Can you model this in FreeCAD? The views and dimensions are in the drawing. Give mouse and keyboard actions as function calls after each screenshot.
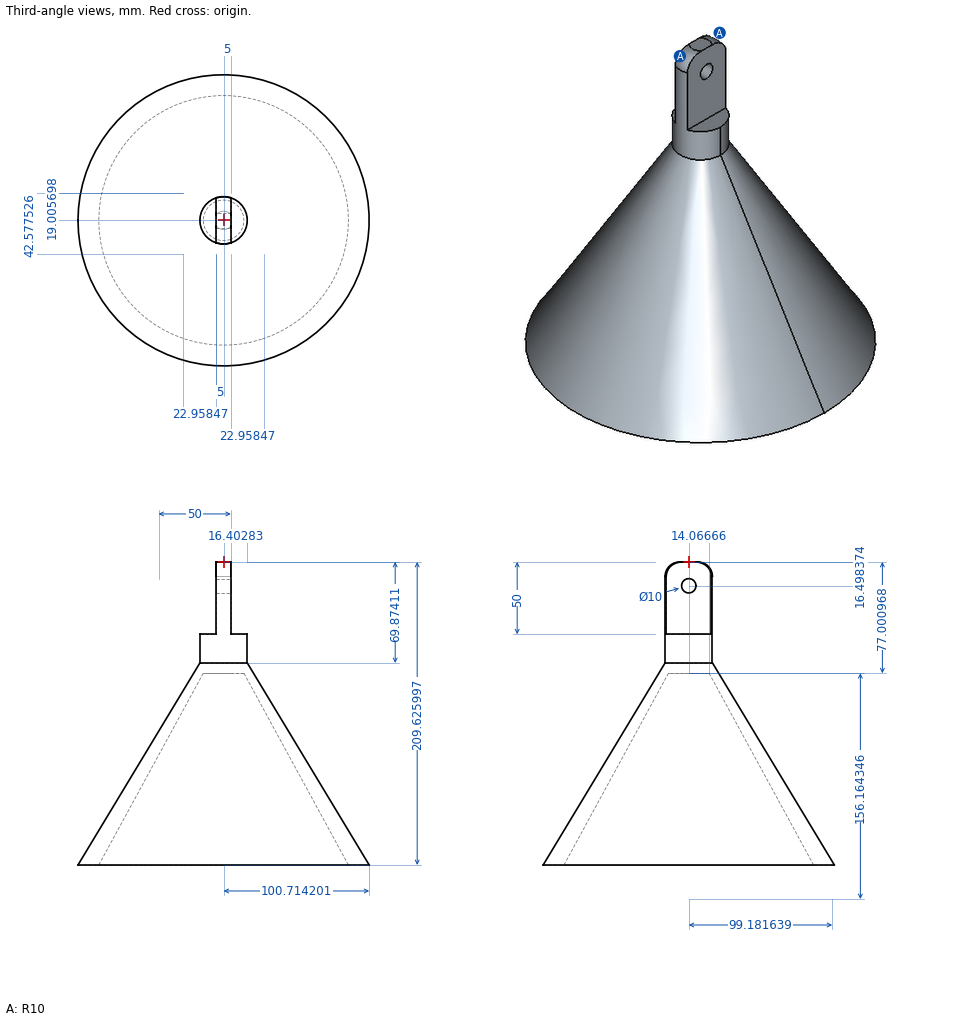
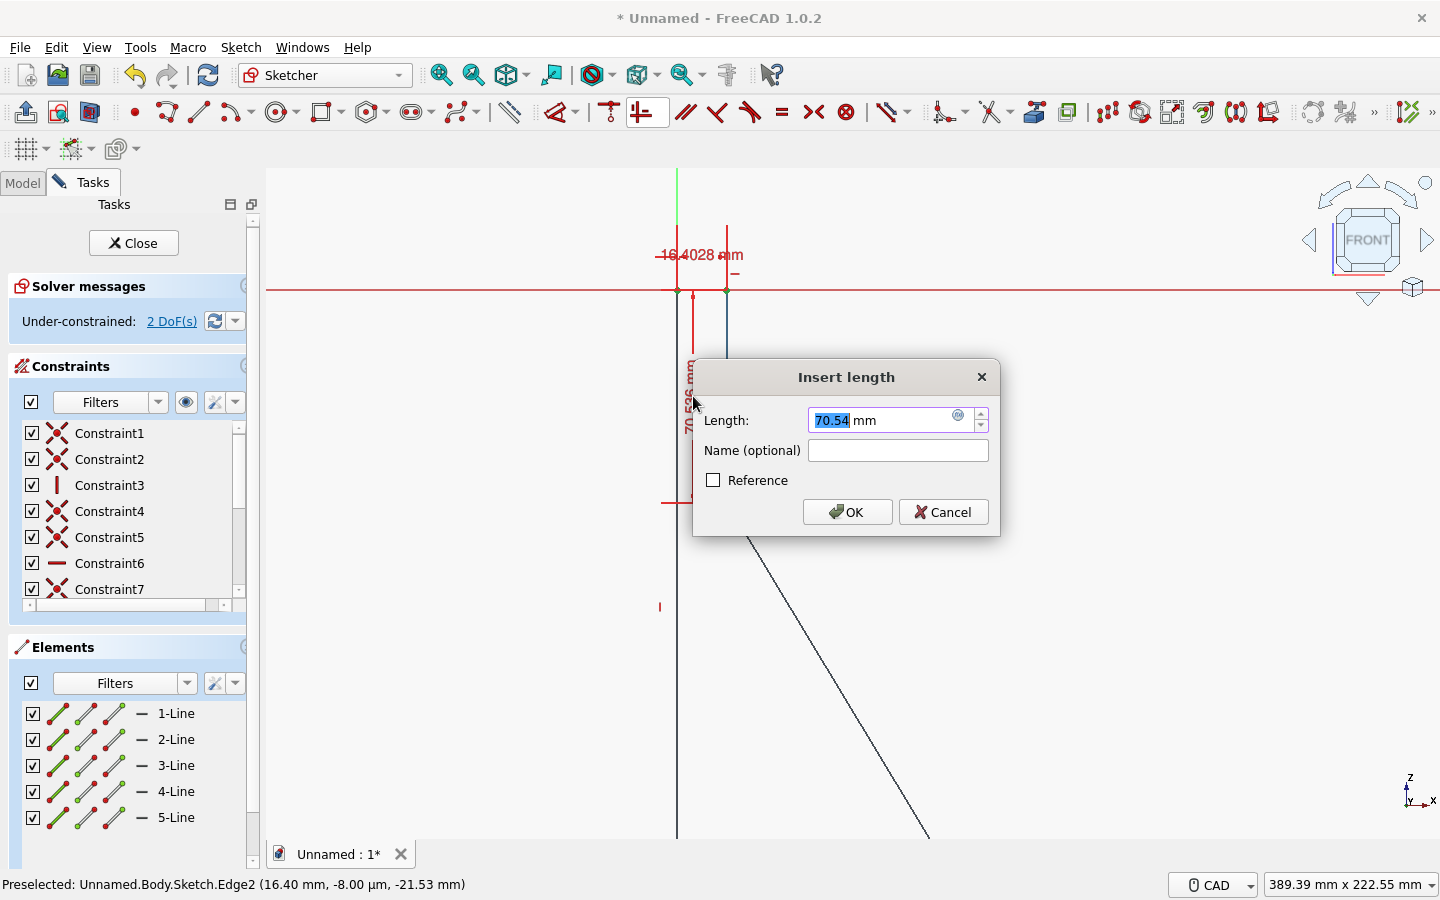
text(69.87411)
key(Return)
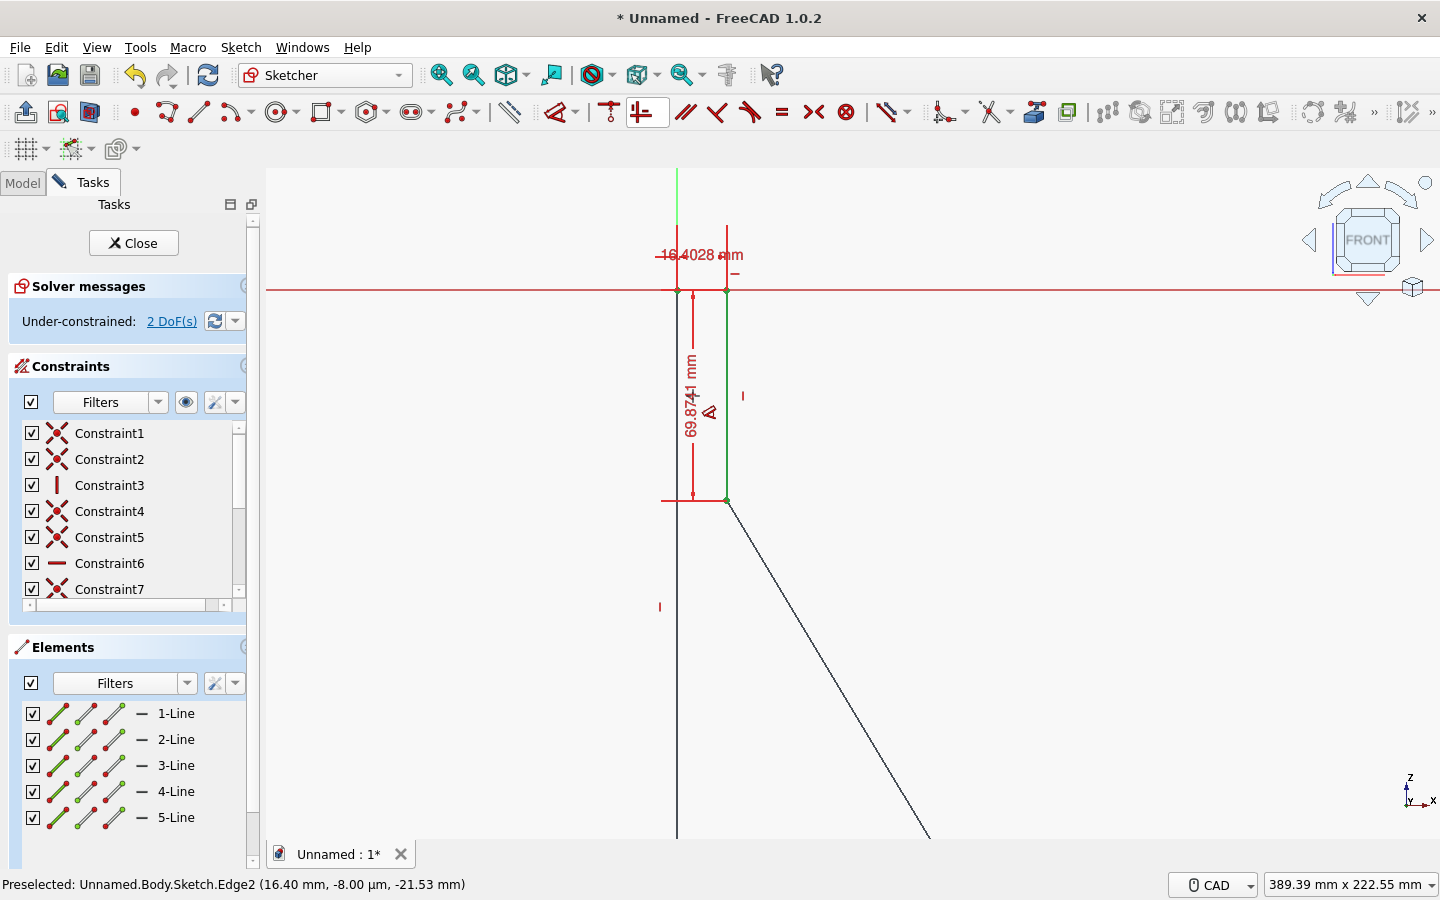
scroll(693, 295, down, 2)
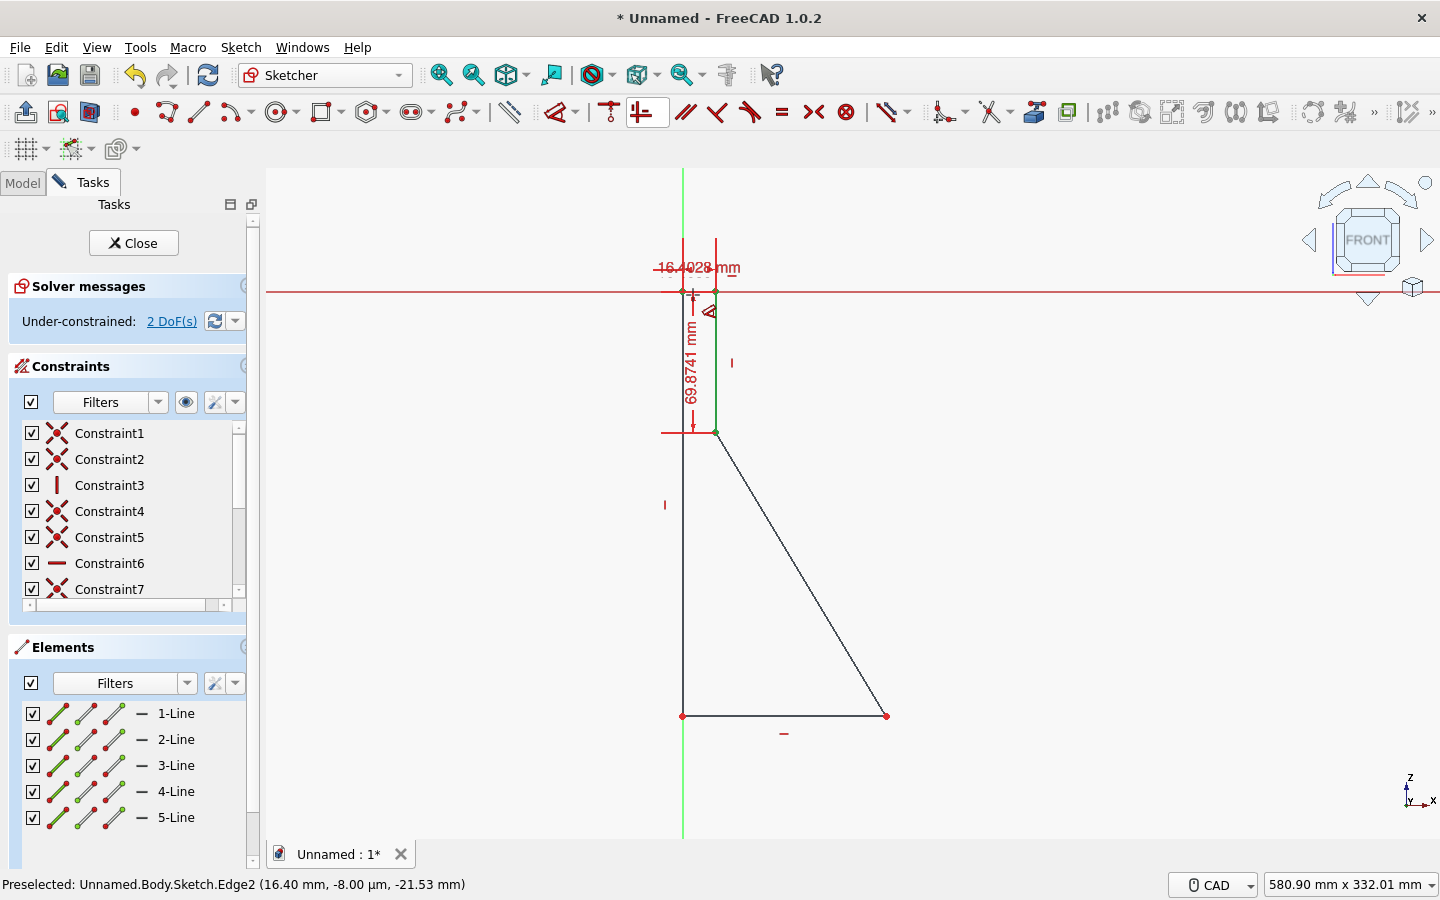
click(825, 716)
click(784, 750)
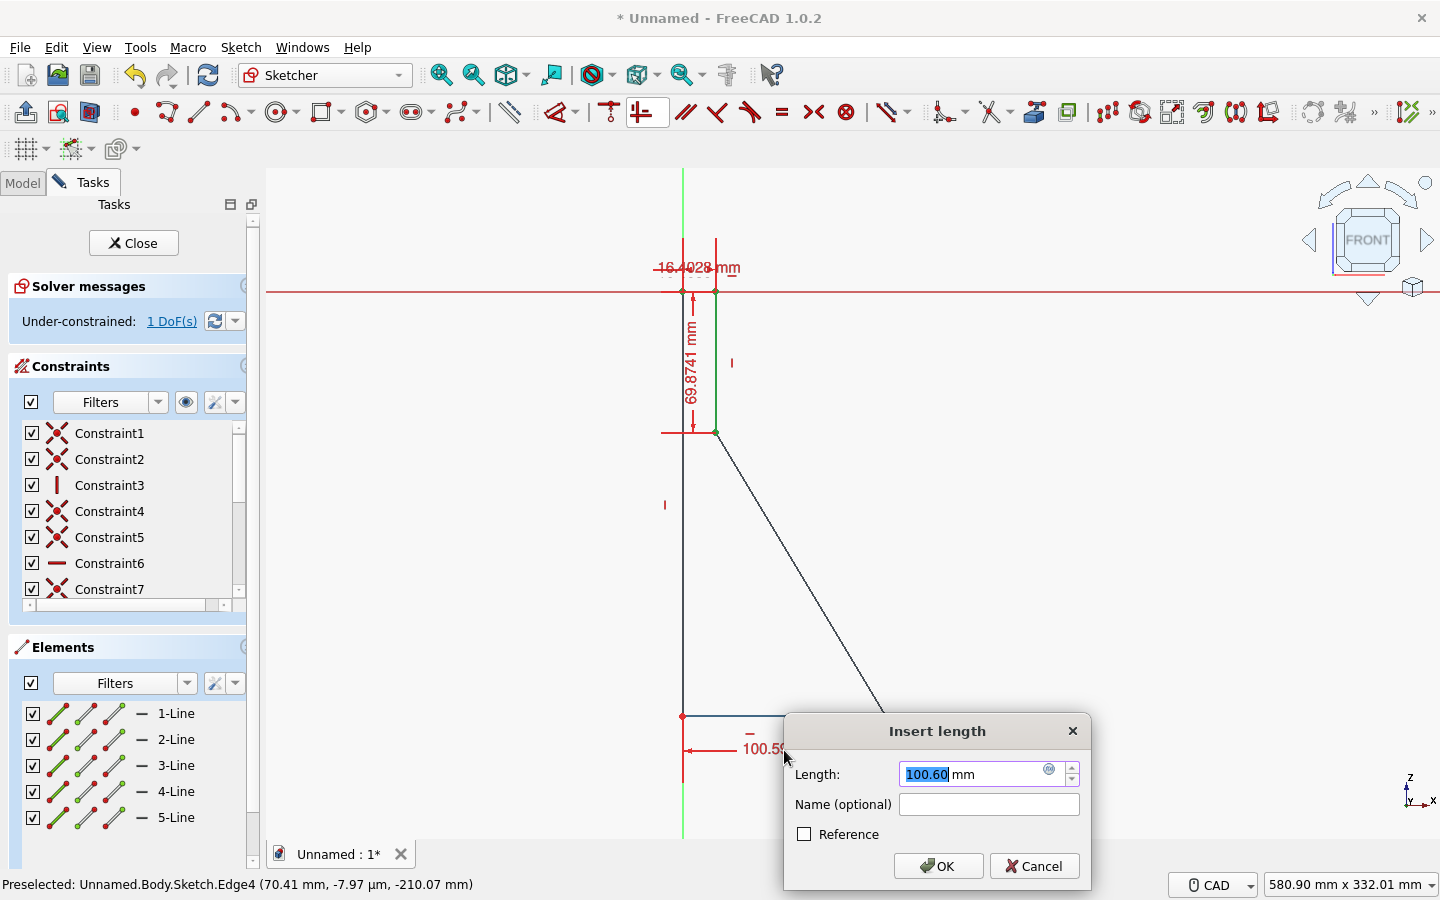
text(100.714201)
key(Return)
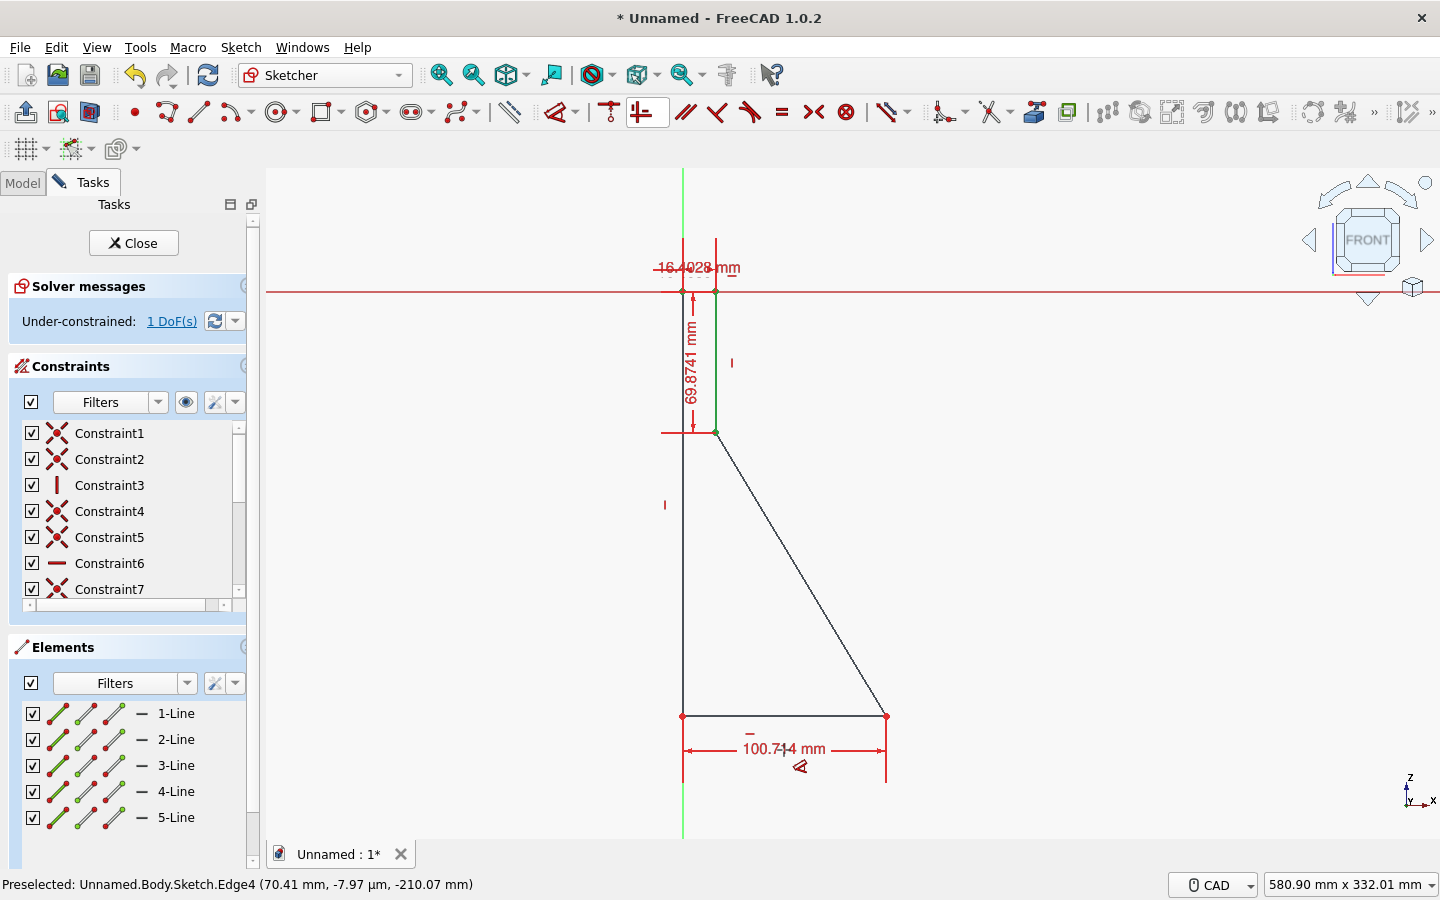
click(683, 589)
click(649, 504)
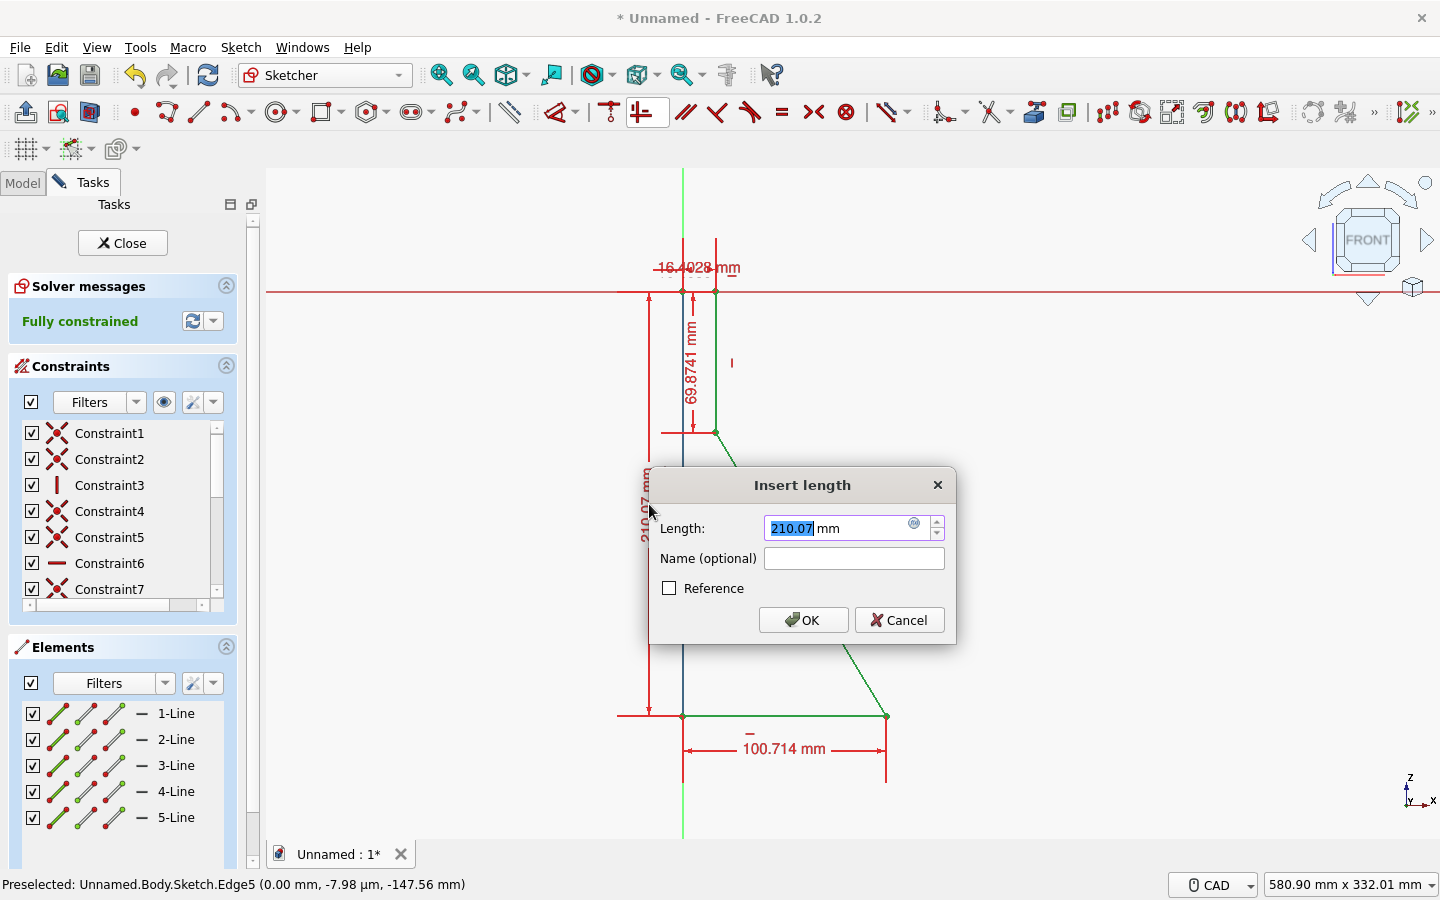
text(209.625997)
key(Return)
key(Escape)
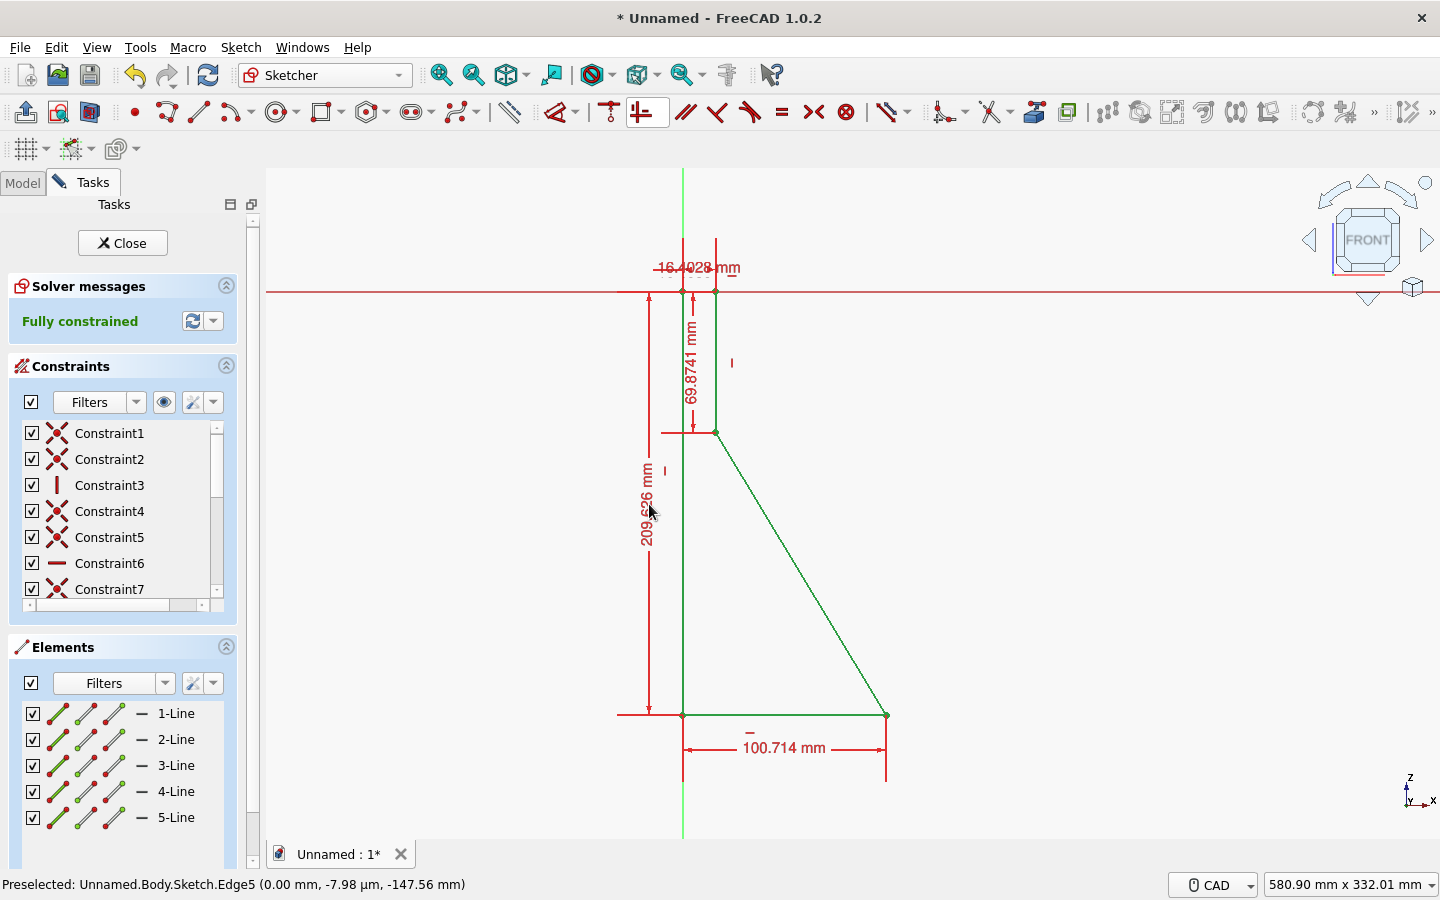
click(123, 243)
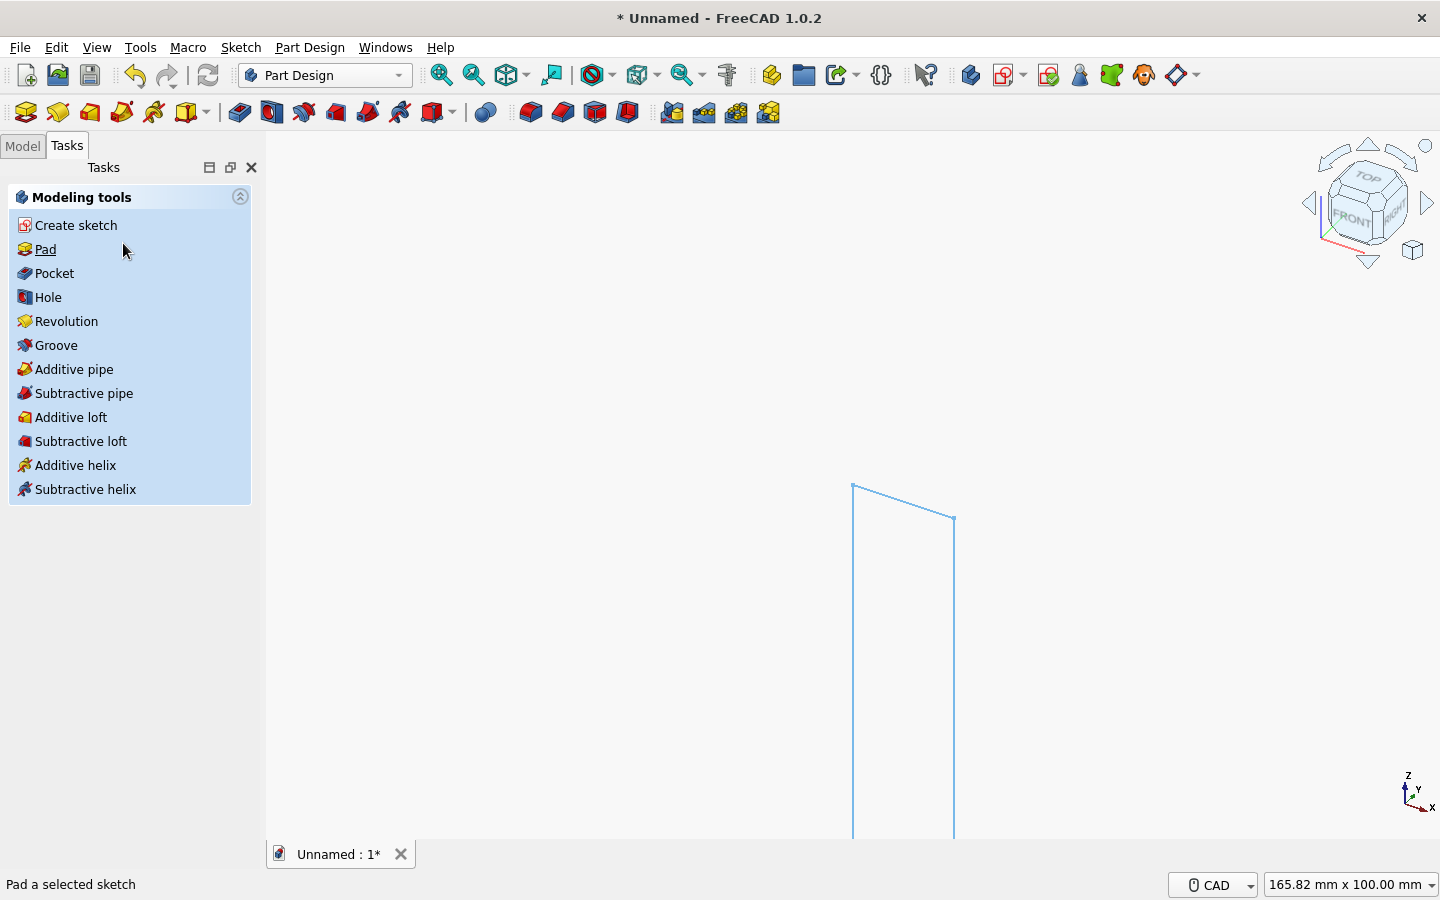
click(58, 112)